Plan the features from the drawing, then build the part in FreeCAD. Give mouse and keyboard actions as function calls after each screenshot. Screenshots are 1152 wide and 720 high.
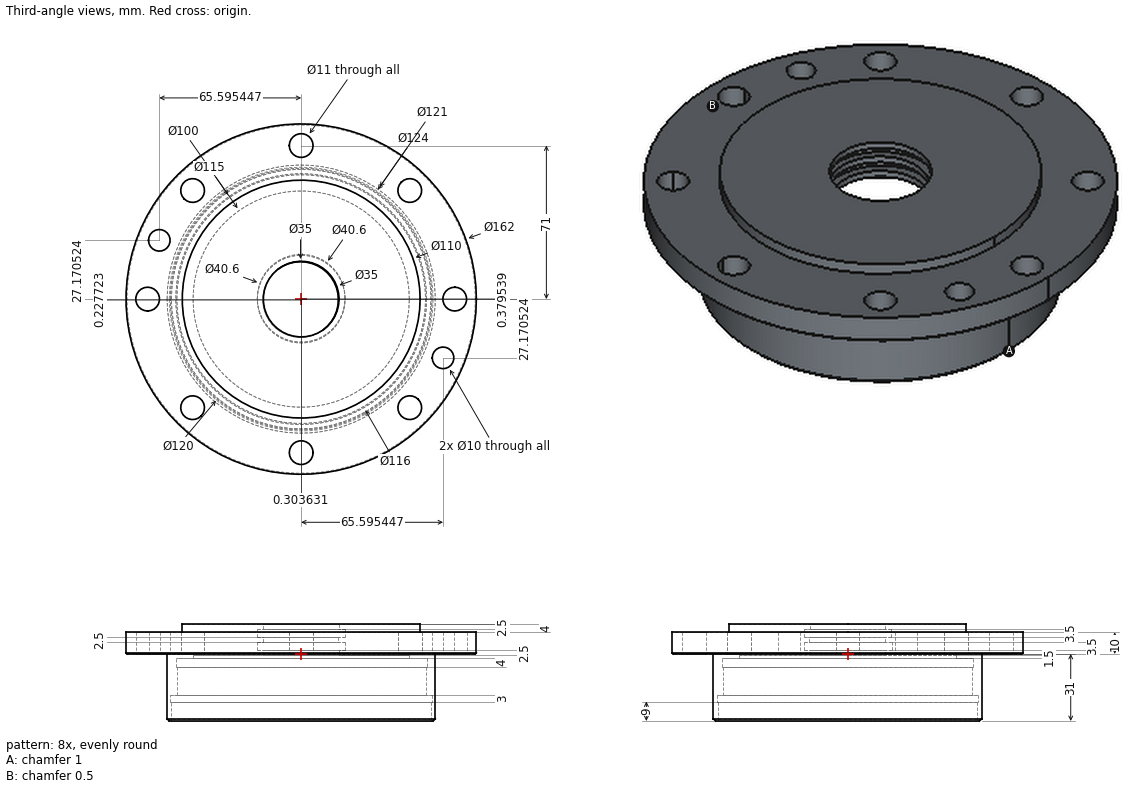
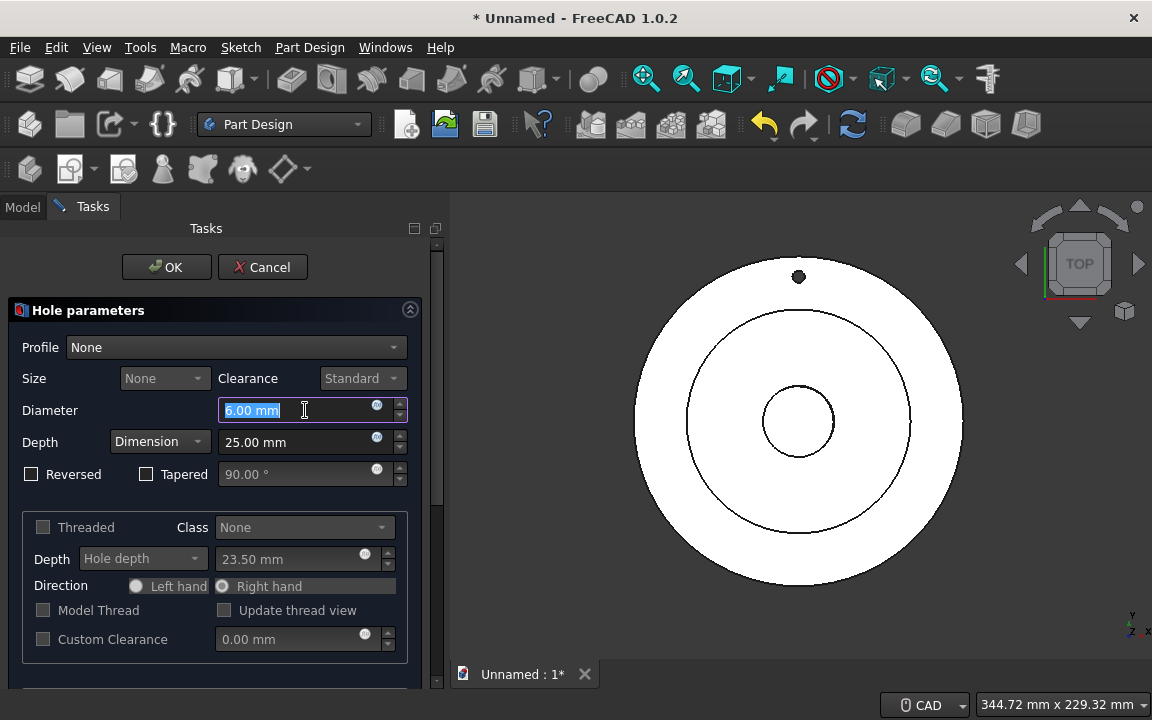
text(11)
key(Tab)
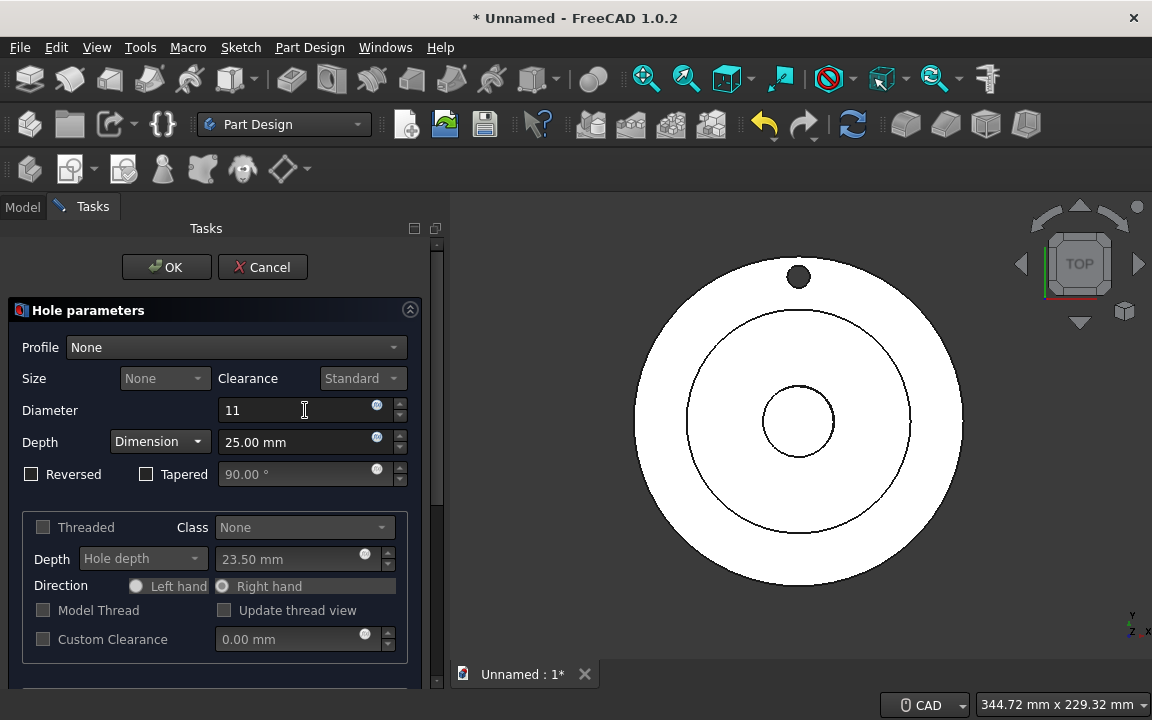
click(161, 442)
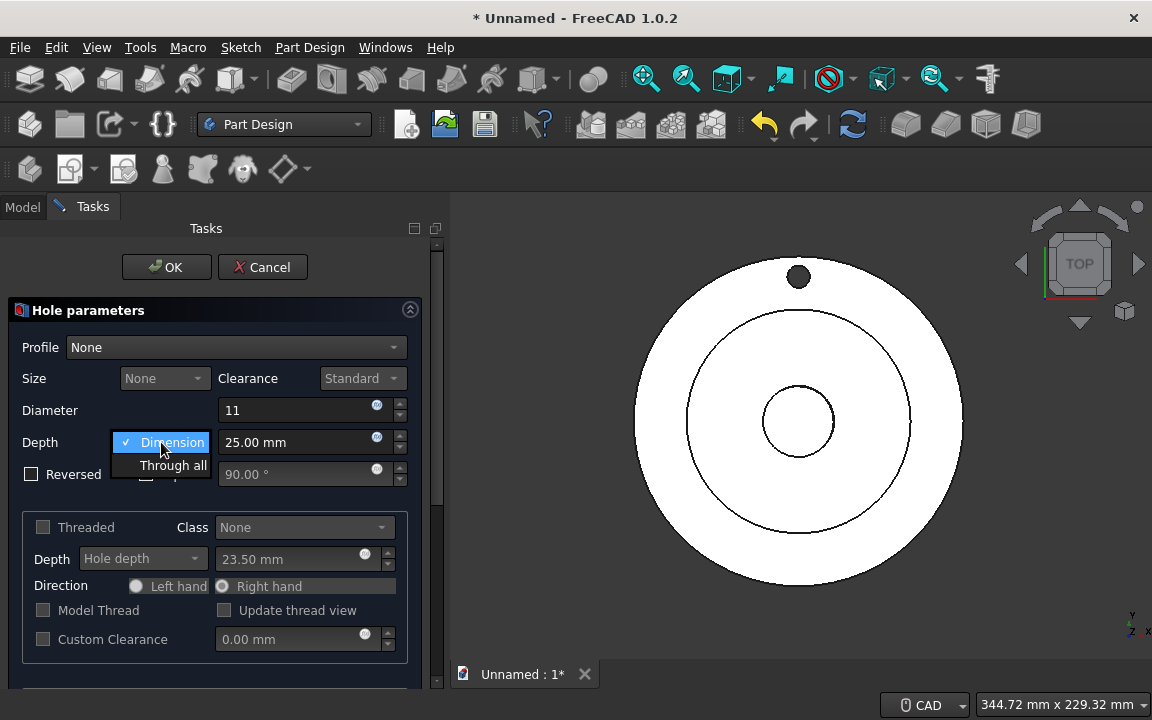
click(160, 466)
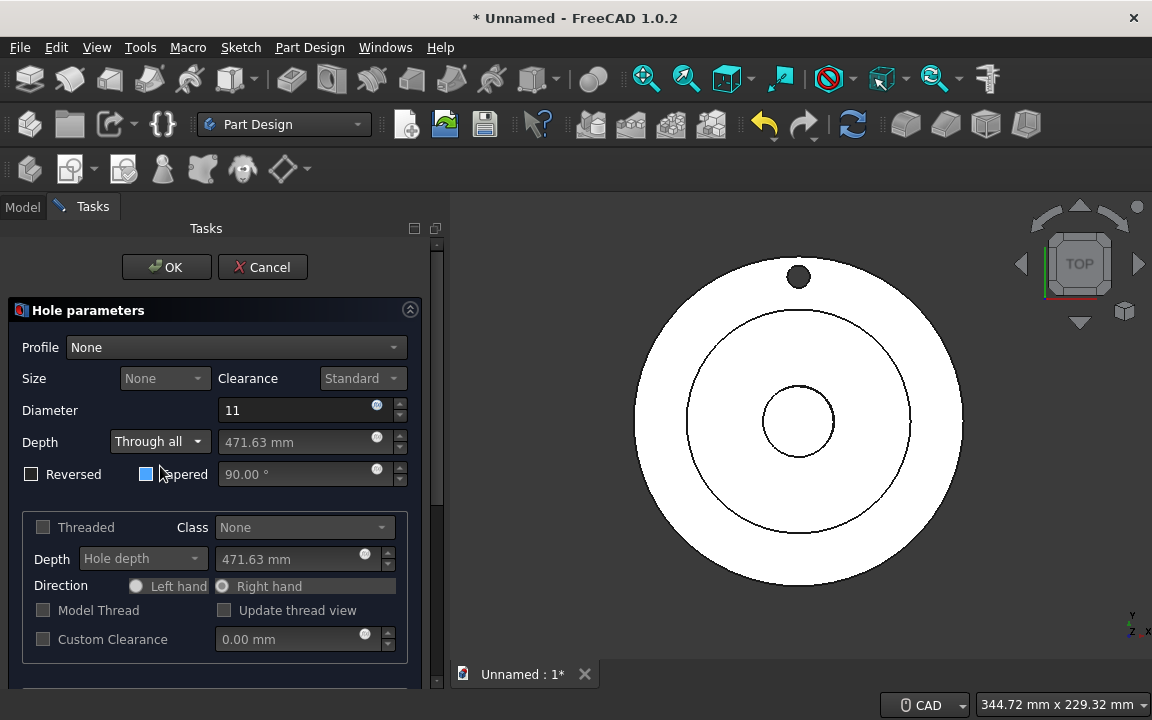
click(167, 267)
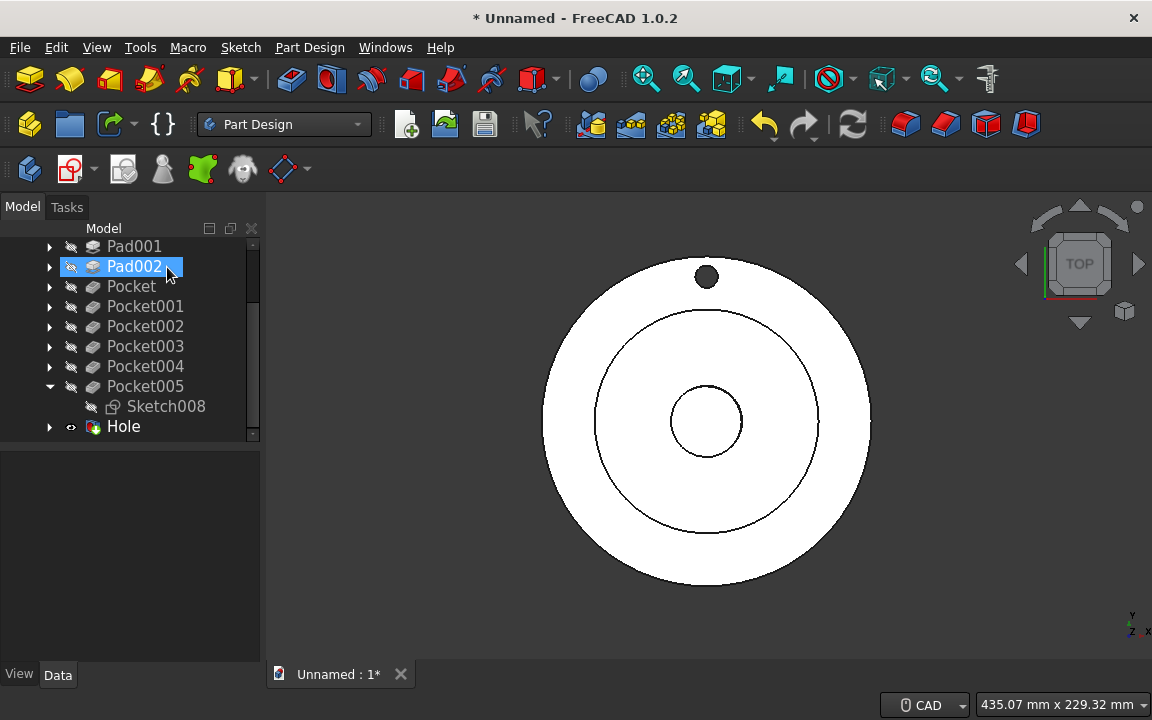
click(116, 427)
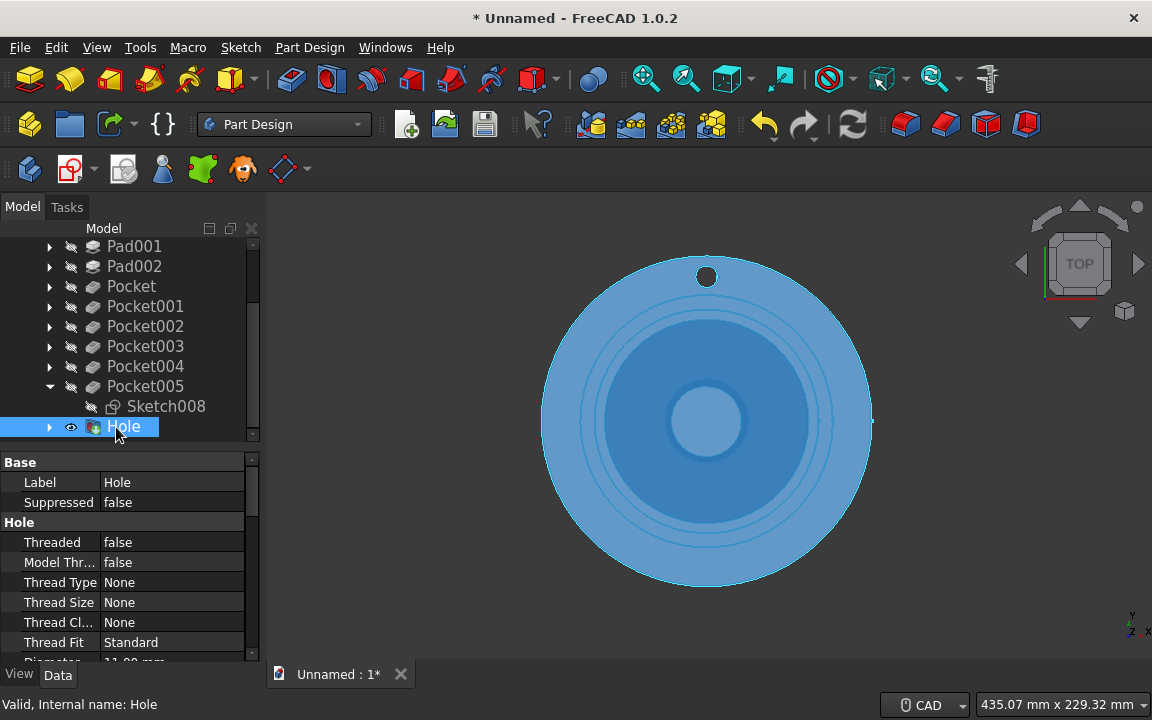
click(672, 124)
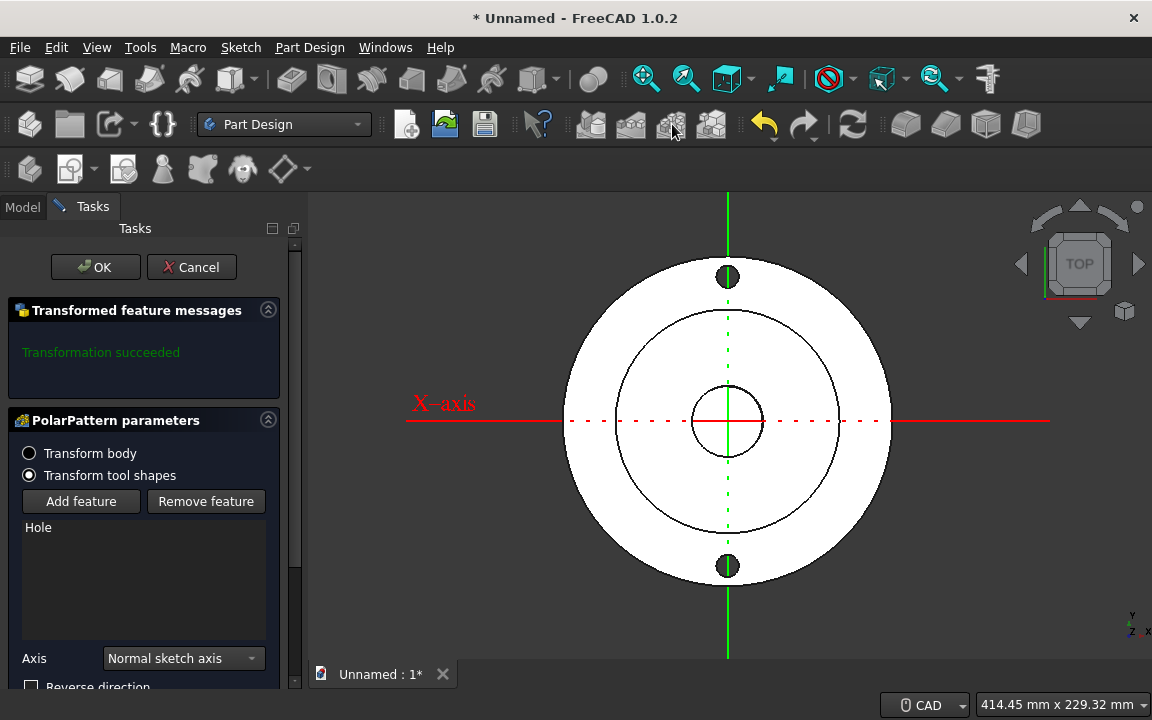
click(184, 658)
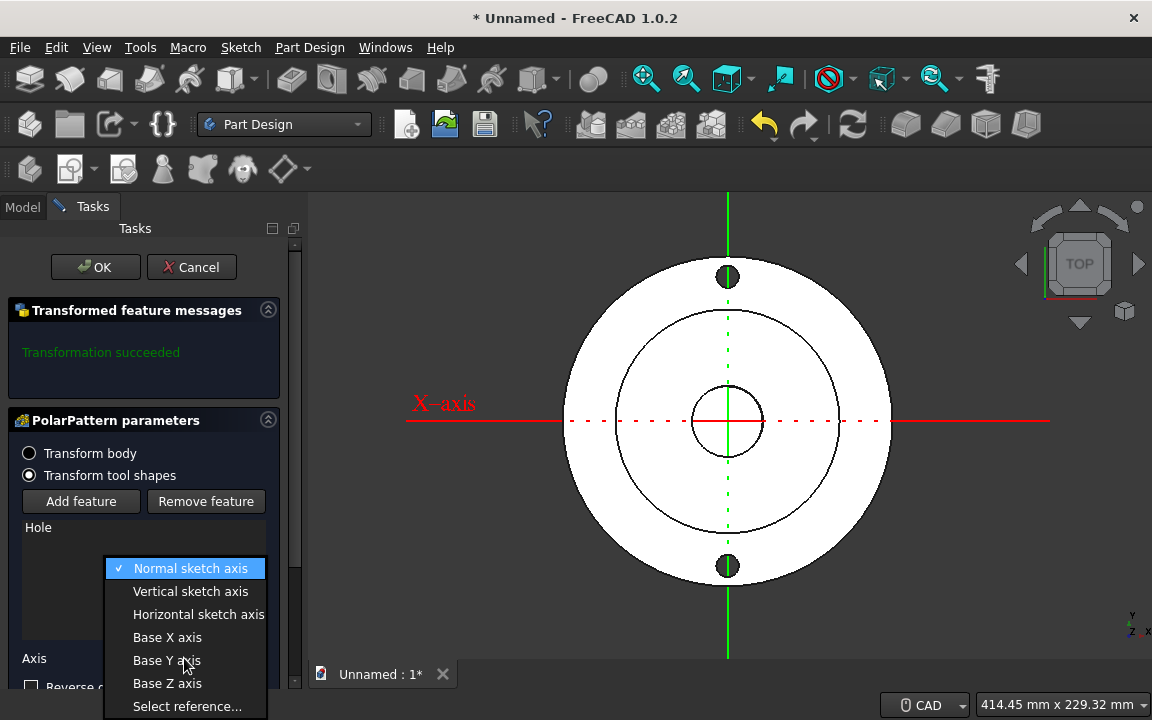
click(184, 684)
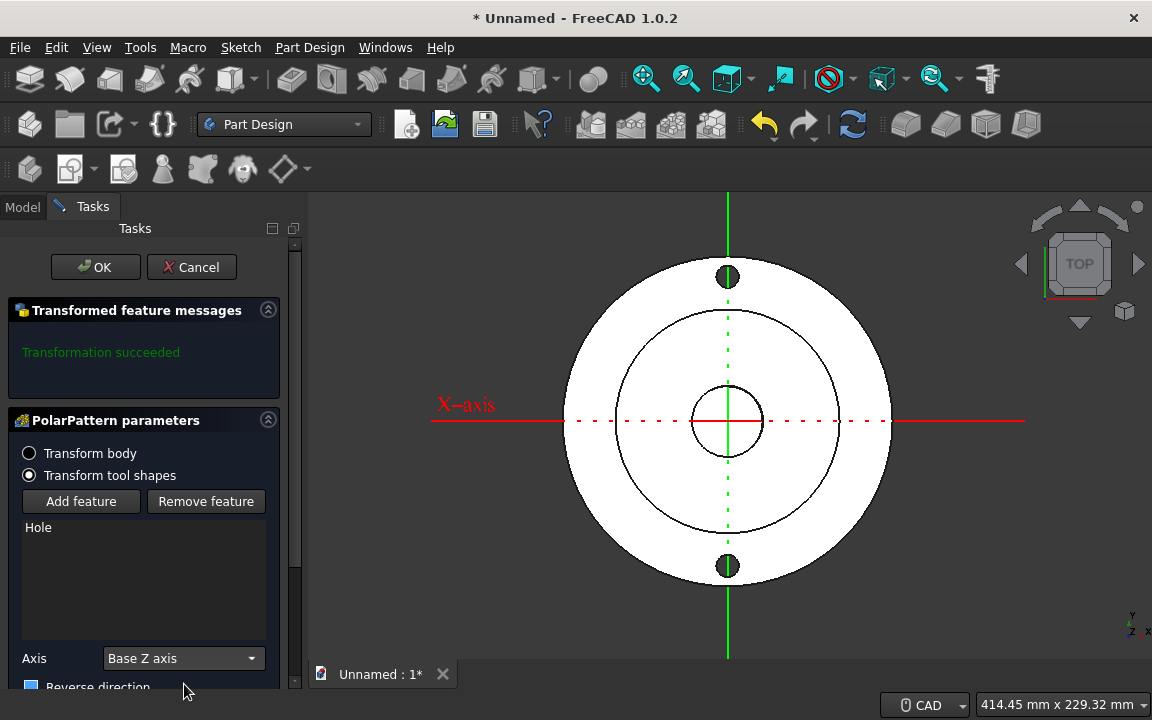
scroll(295, 463, down, 3)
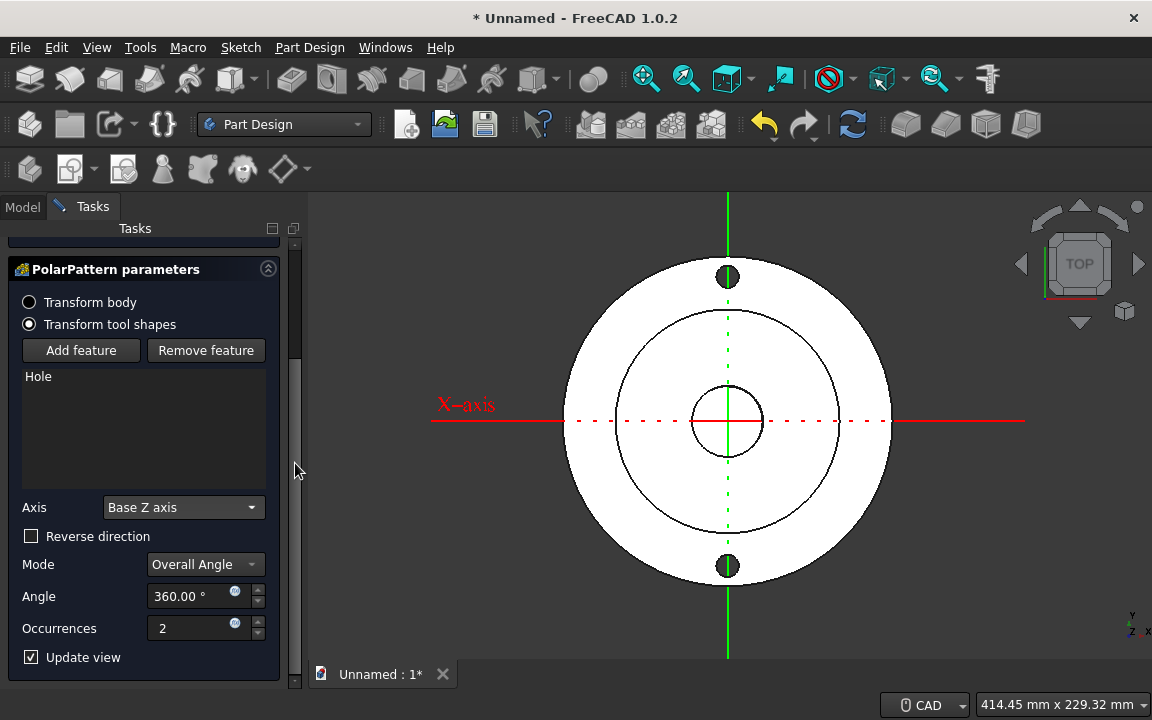
triple_click(198, 628)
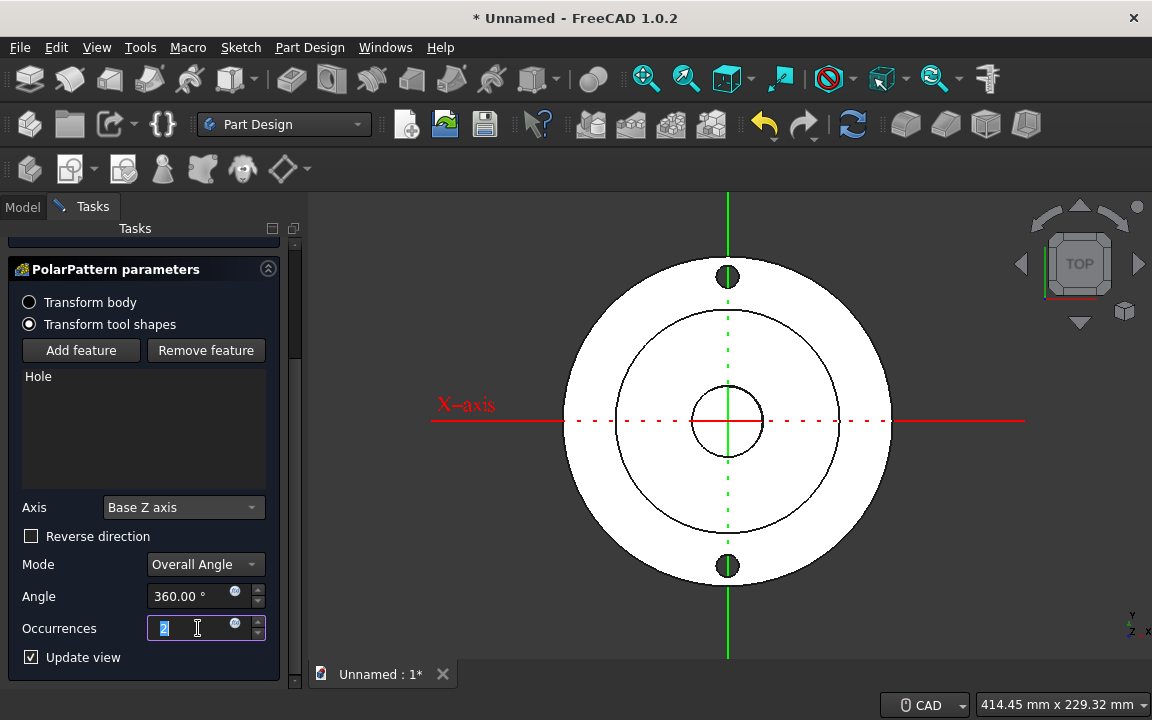
text(8)
key(Tab)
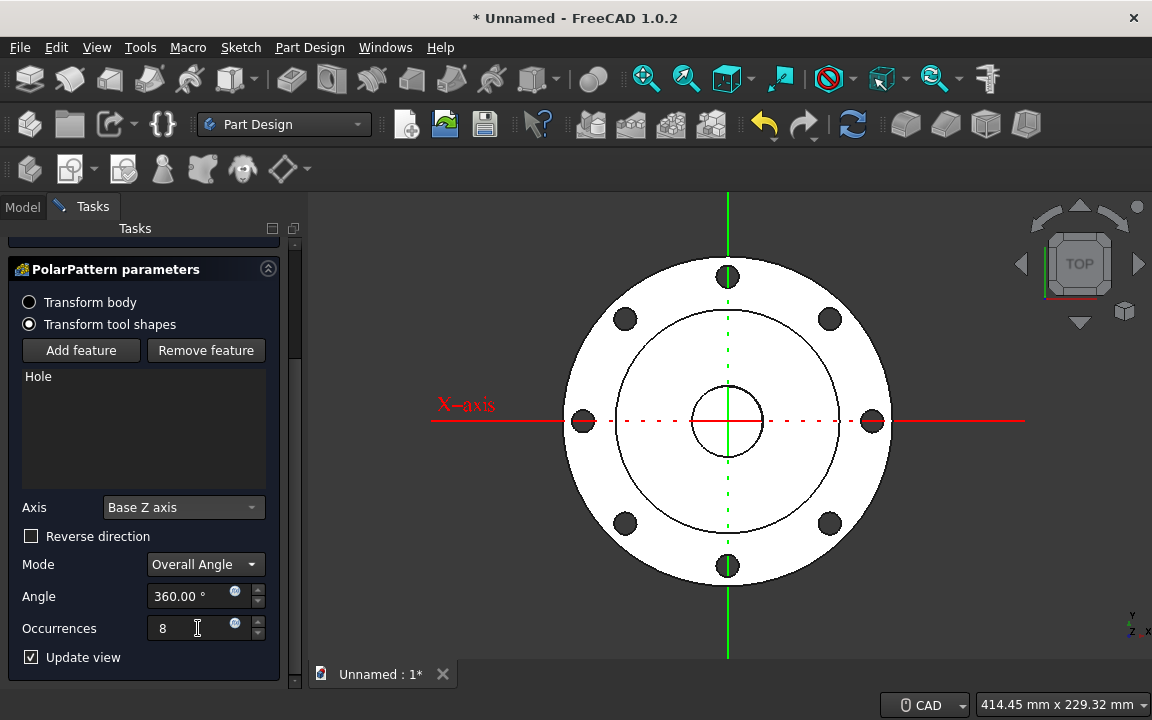
scroll(295, 463, up, 4)